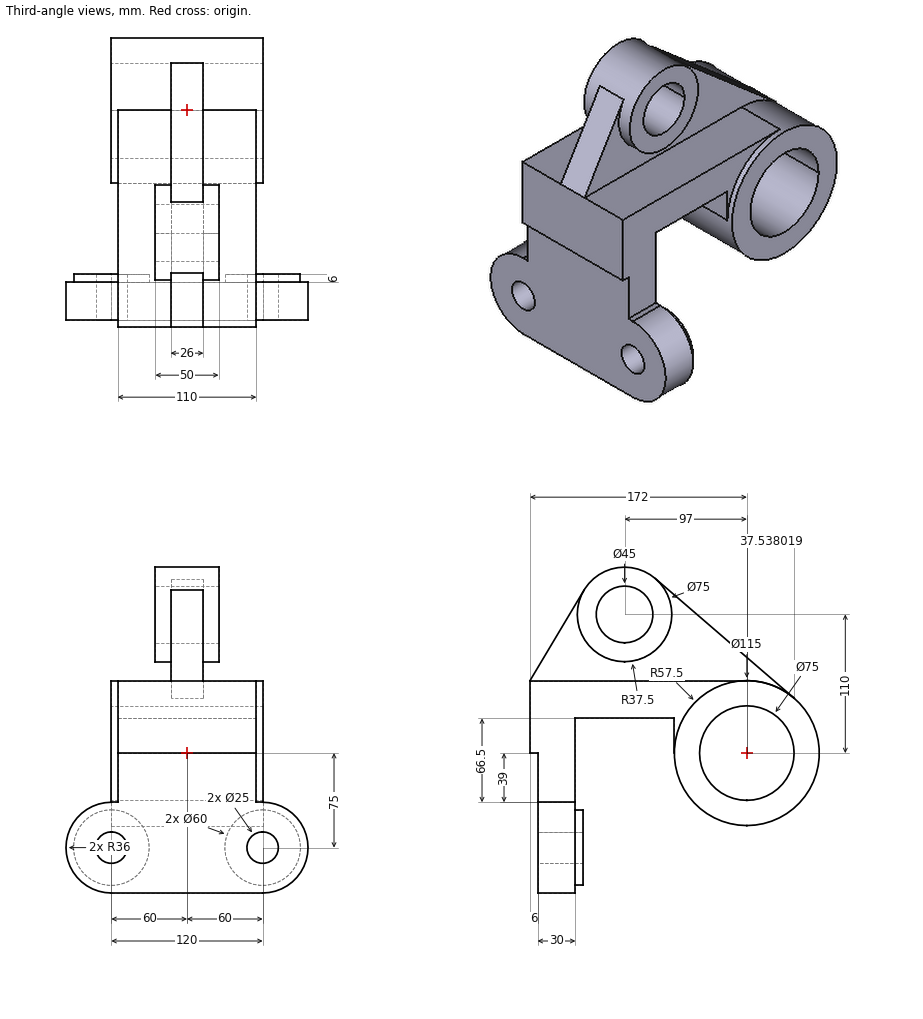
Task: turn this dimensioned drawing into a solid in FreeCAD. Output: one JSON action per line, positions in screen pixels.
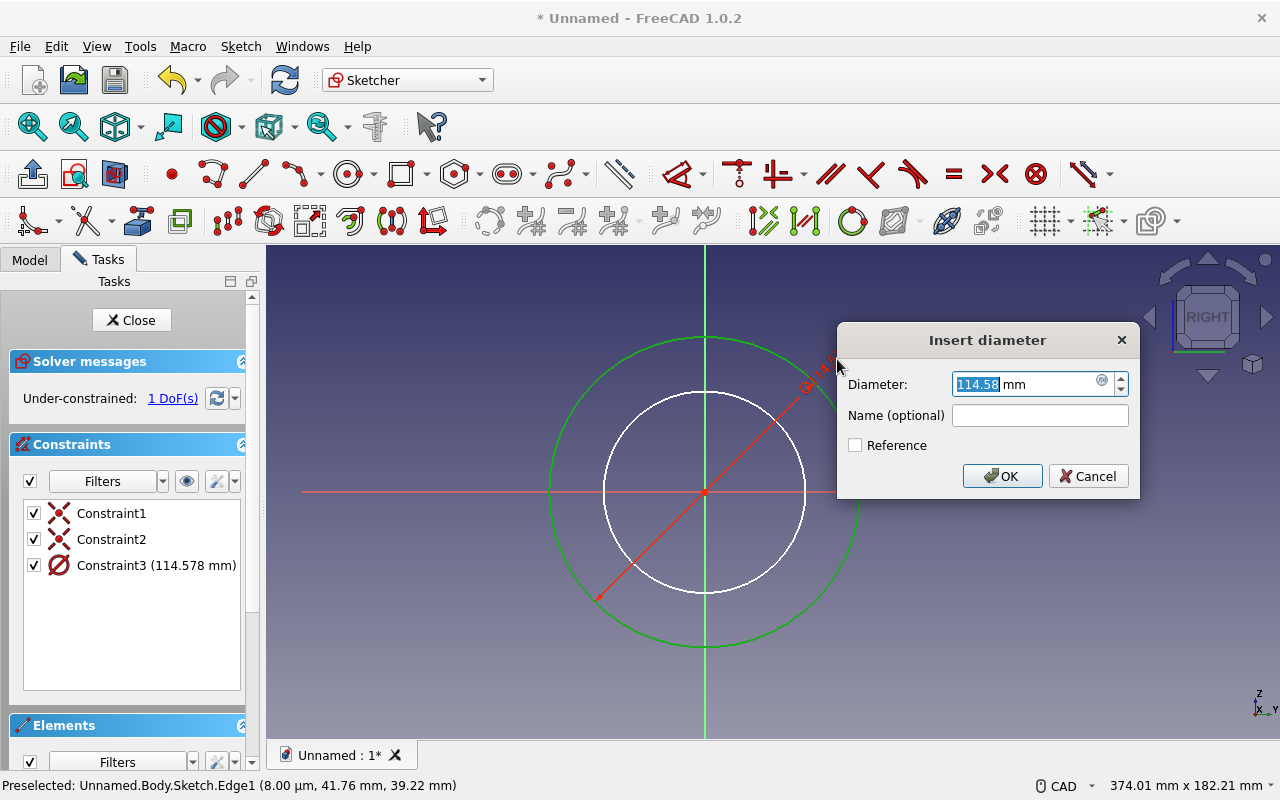
{"action": "type", "text": "115"}
{"action": "key", "text": "Return"}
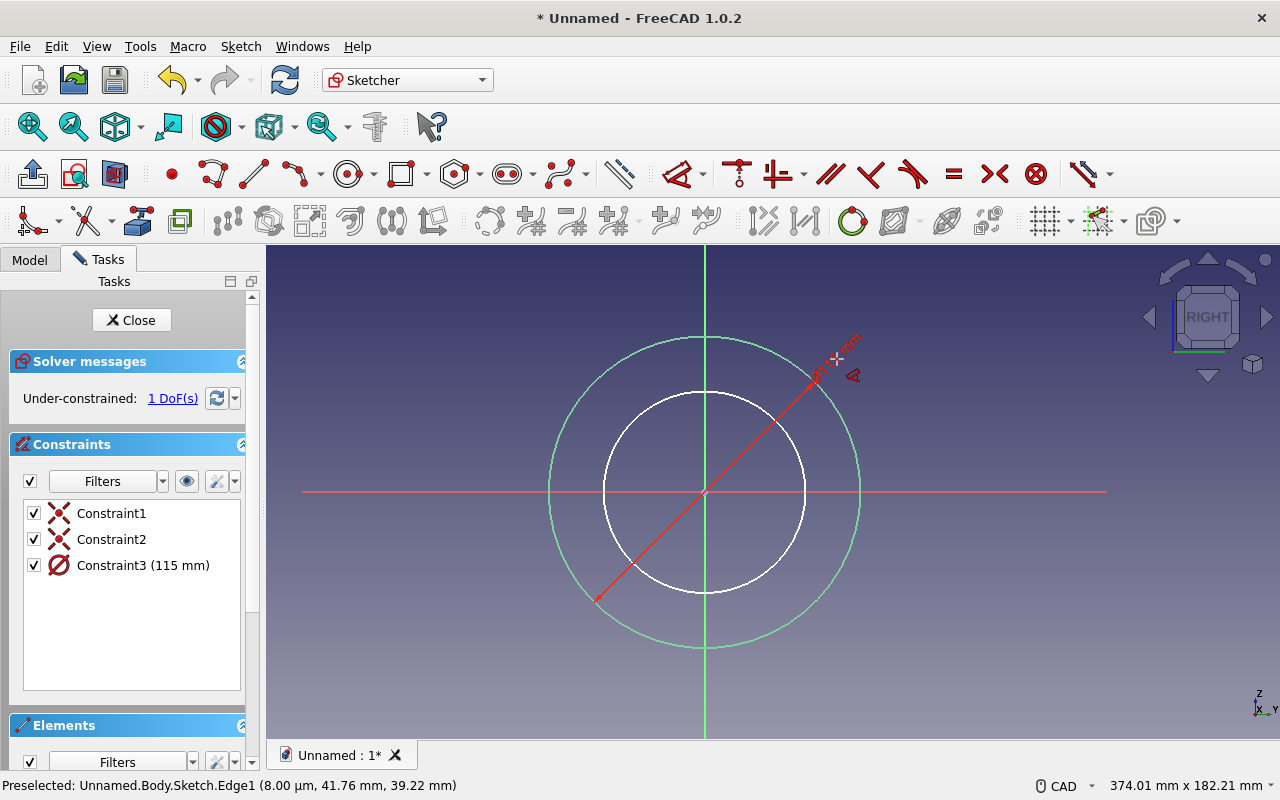
{"action": "left_click", "coordinate": [776, 421]}
{"action": "left_click", "coordinate": [799, 398]}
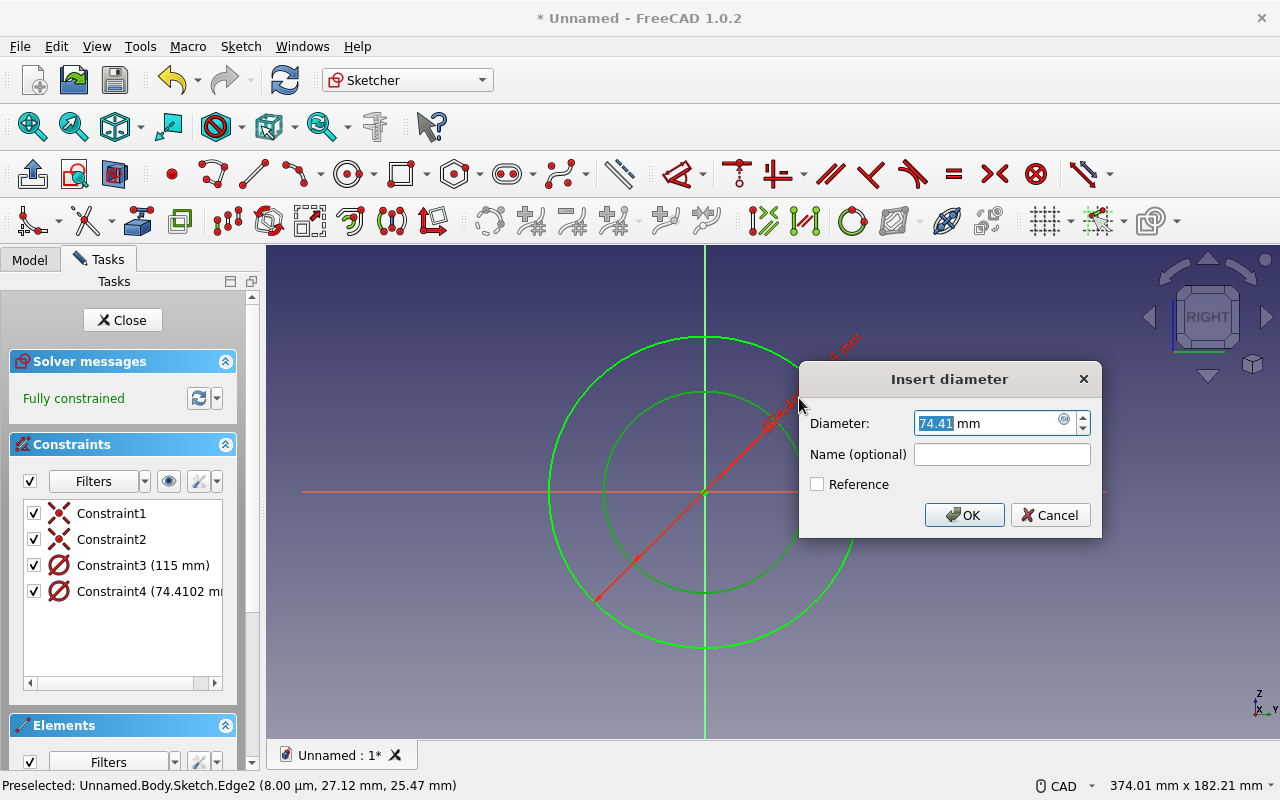
{"action": "type", "text": "75"}
{"action": "key", "text": "Return"}
{"action": "key", "text": "Escape"}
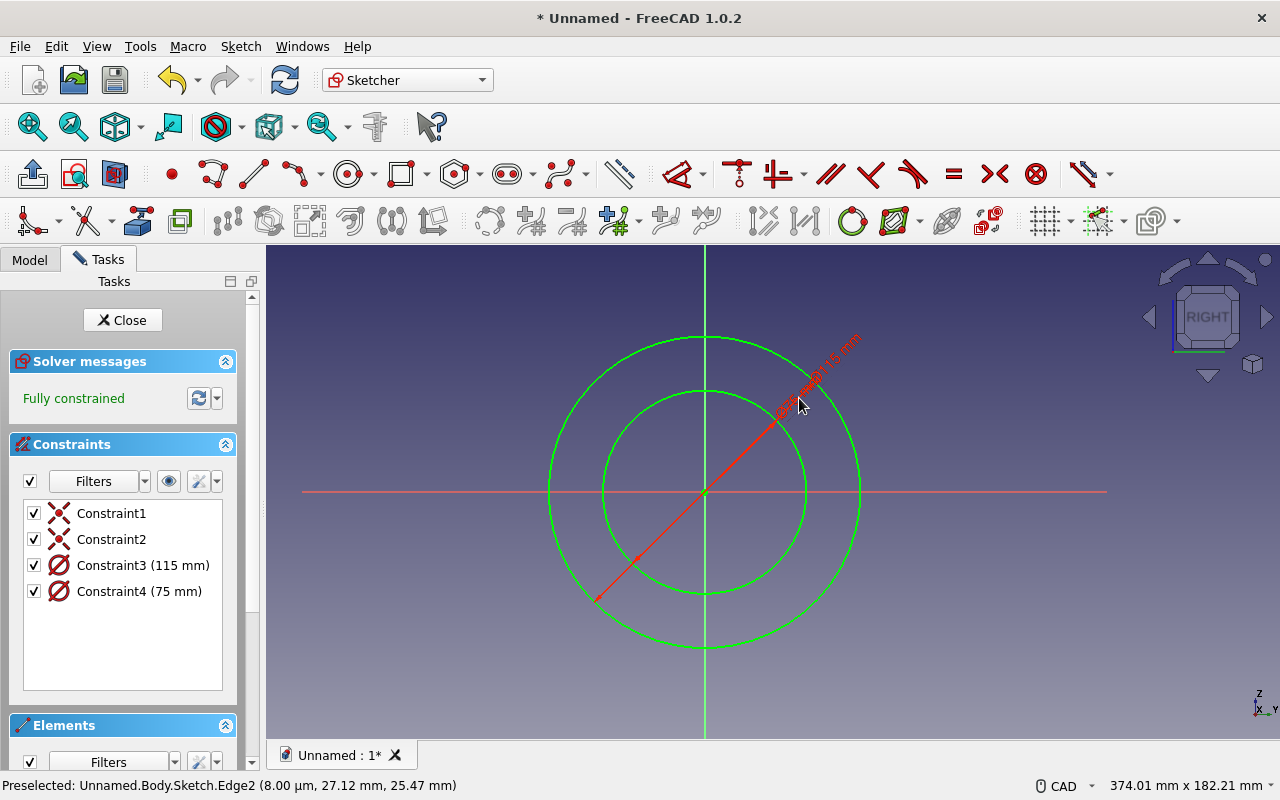
{"action": "left_click", "coordinate": [123, 320]}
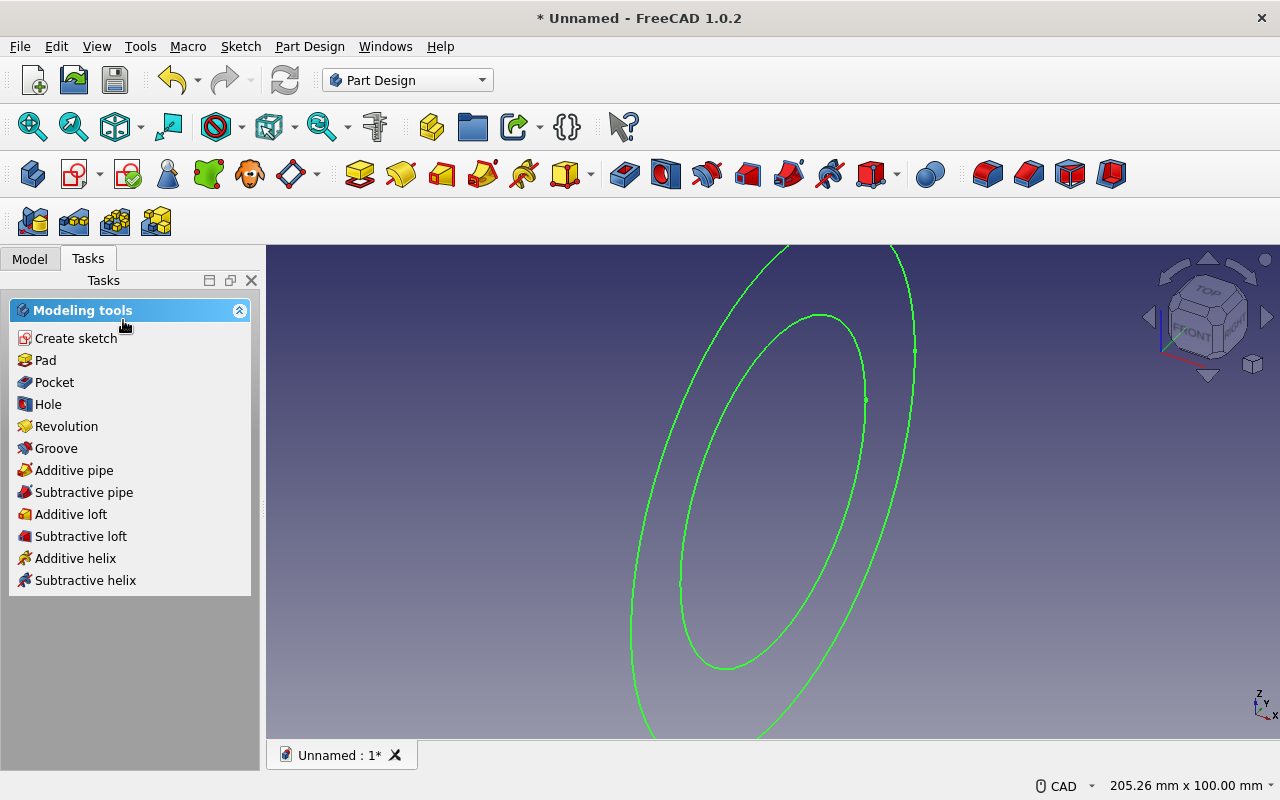
{"action": "left_click", "coordinate": [360, 174]}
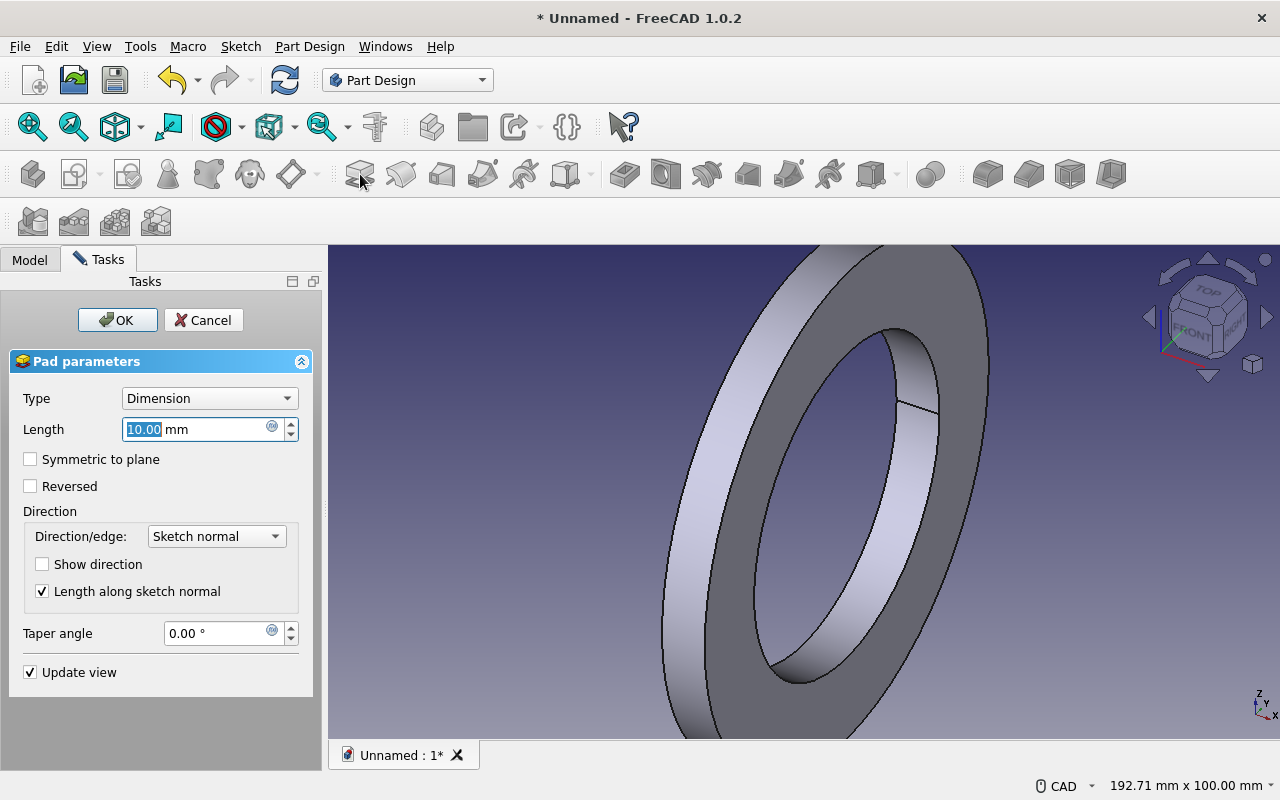
{"action": "type", "text": "120"}
{"action": "key", "text": "Tab"}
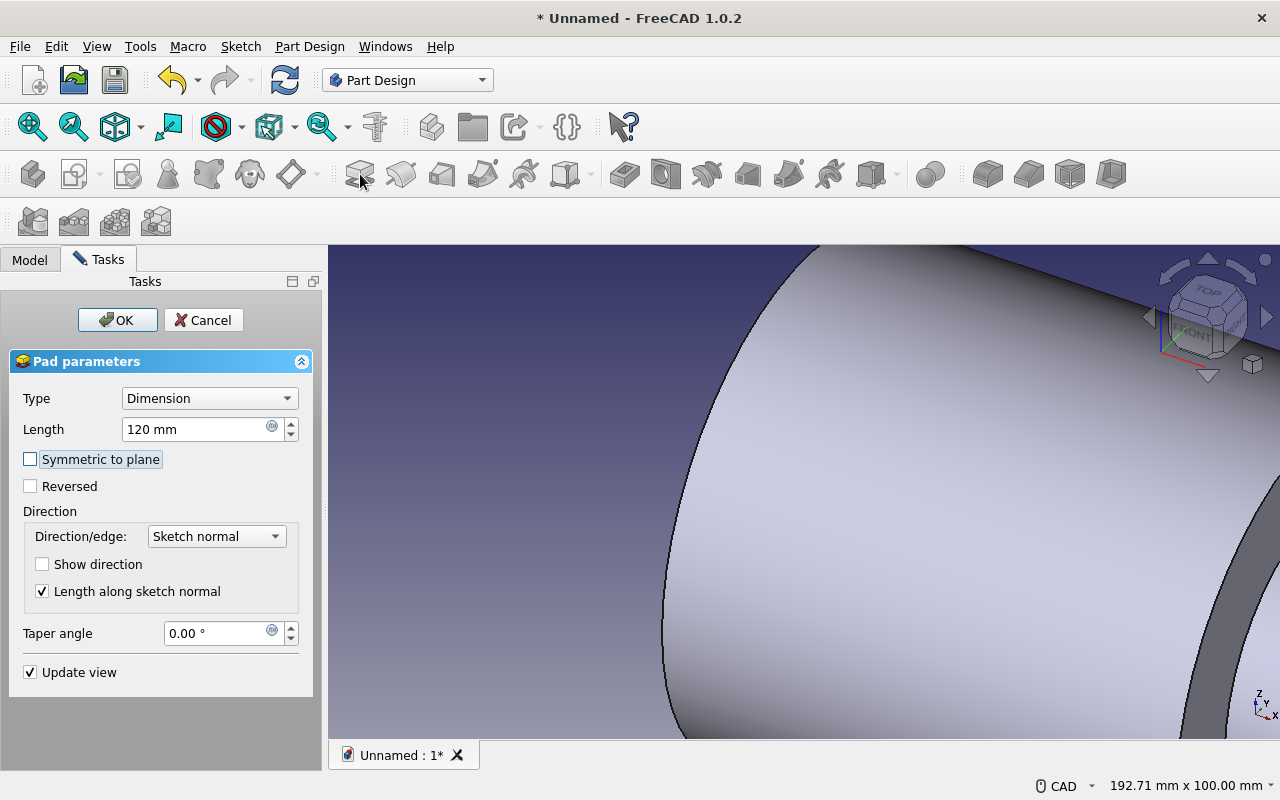
{"action": "left_click", "coordinate": [31, 459]}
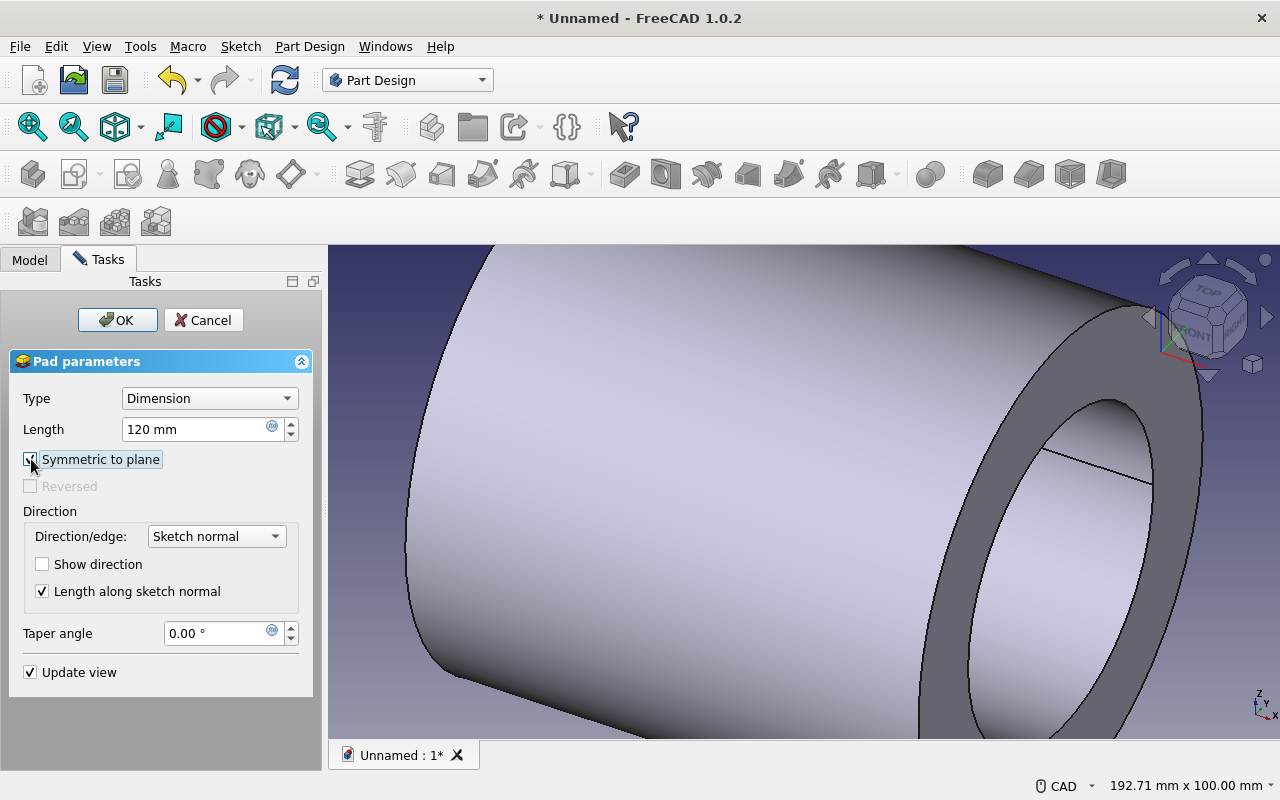
{"action": "left_click", "coordinate": [118, 320]}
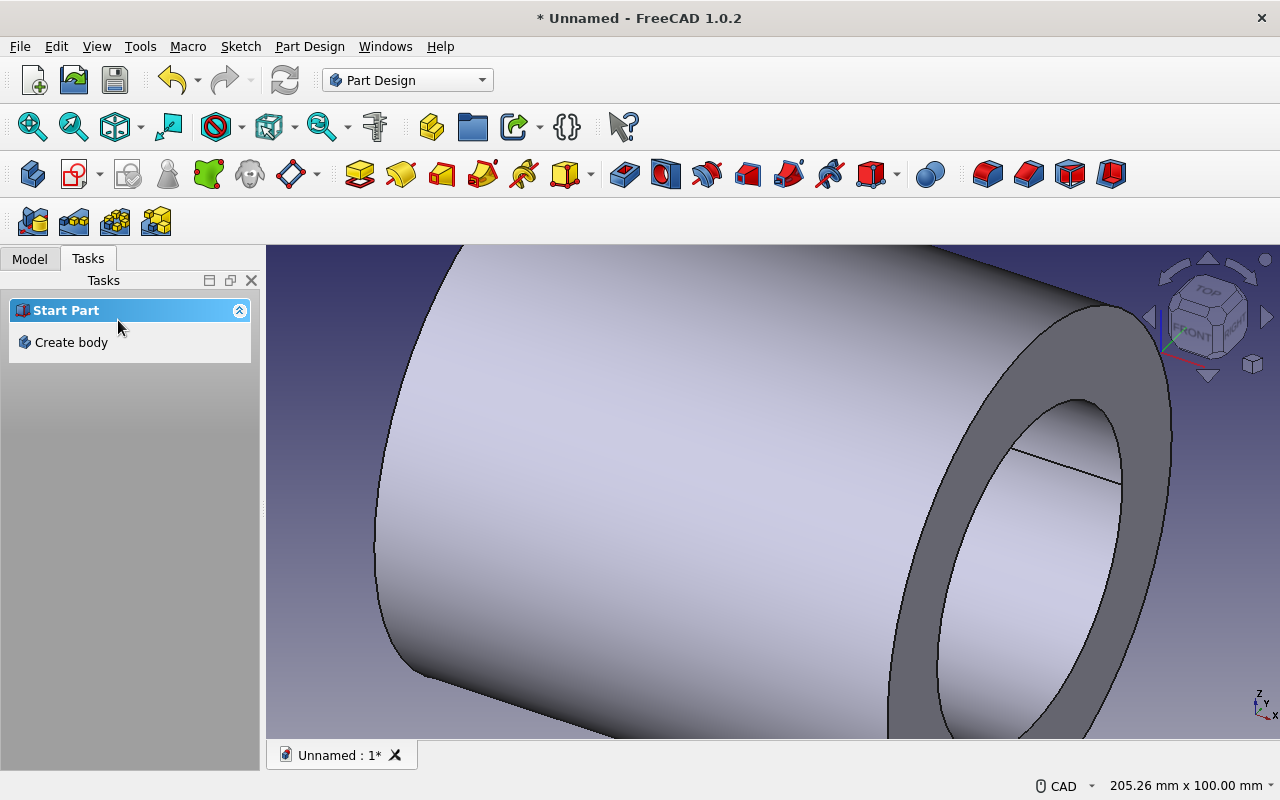
{"action": "key", "text": "v f"}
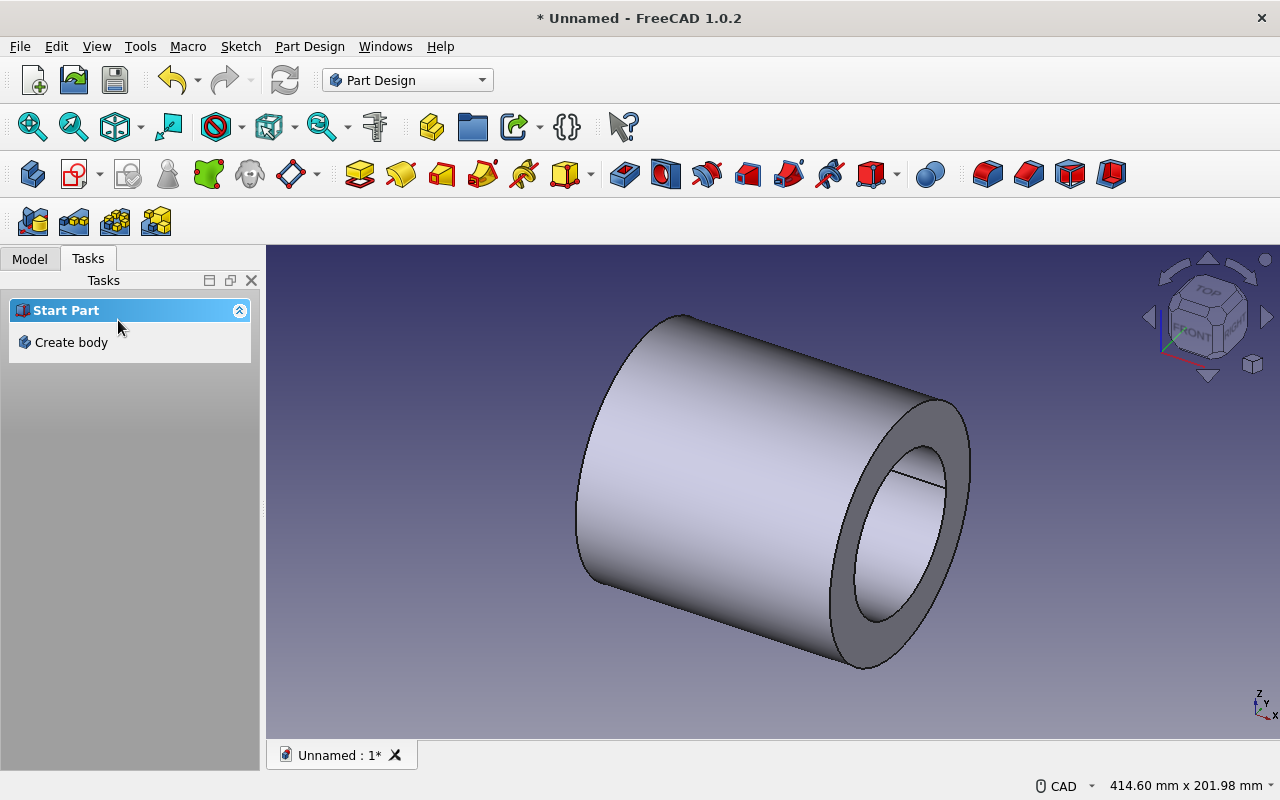
{"action": "left_click", "coordinate": [33, 174]}